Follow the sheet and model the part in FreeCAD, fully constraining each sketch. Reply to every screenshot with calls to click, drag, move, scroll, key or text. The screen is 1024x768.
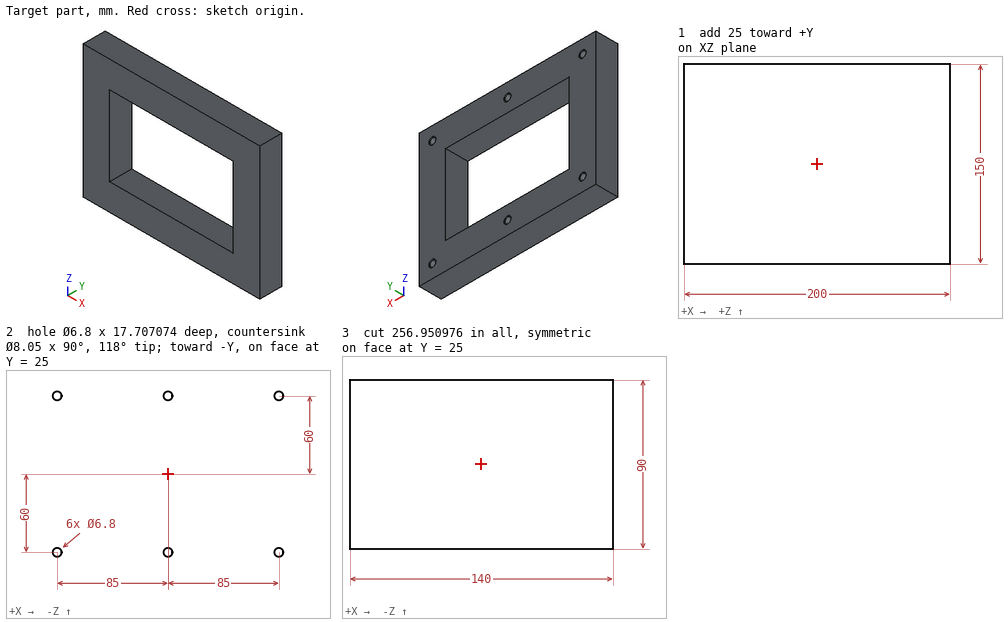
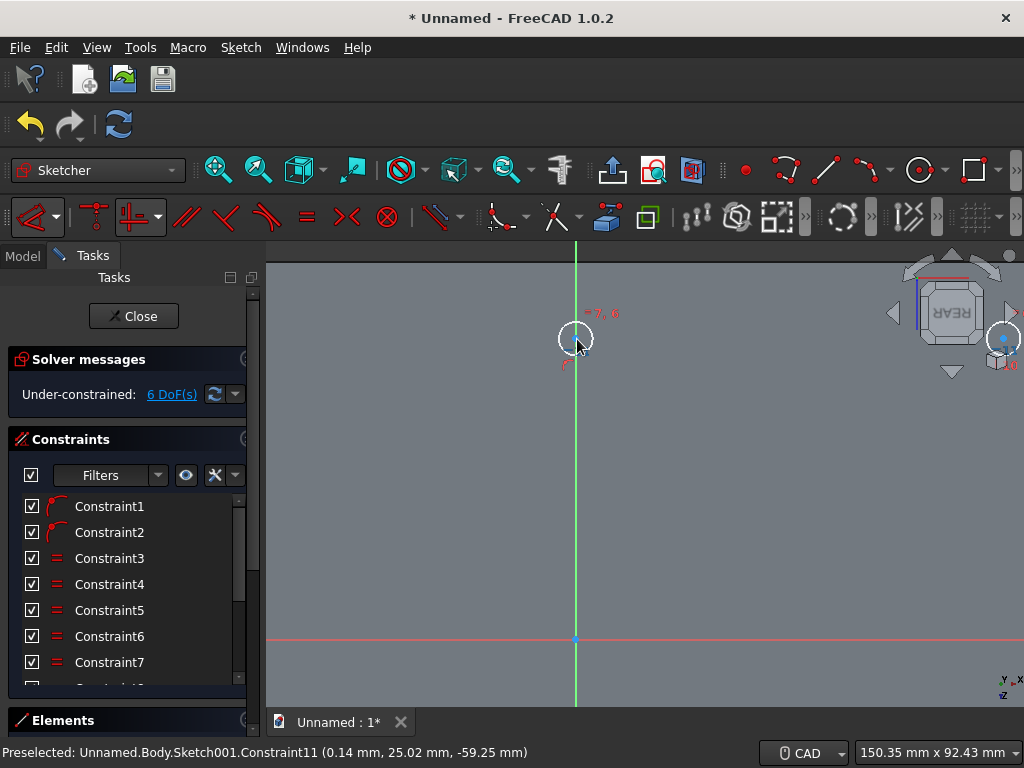
click(576, 339)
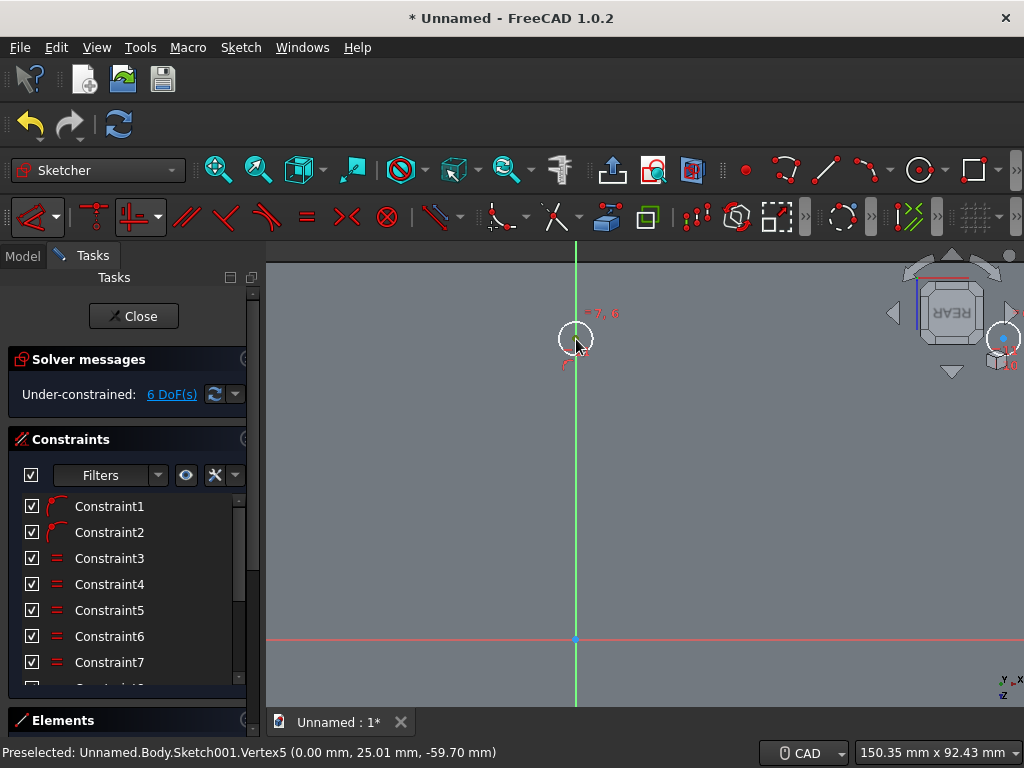
scroll(577, 339, down, 4)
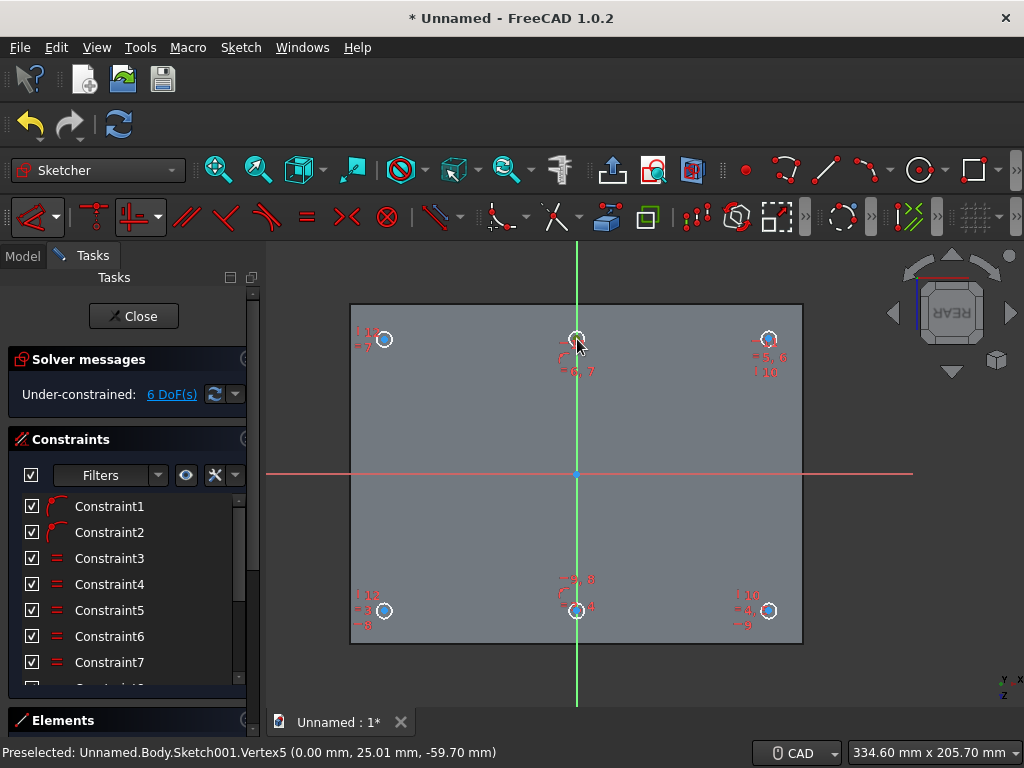
click(384, 339)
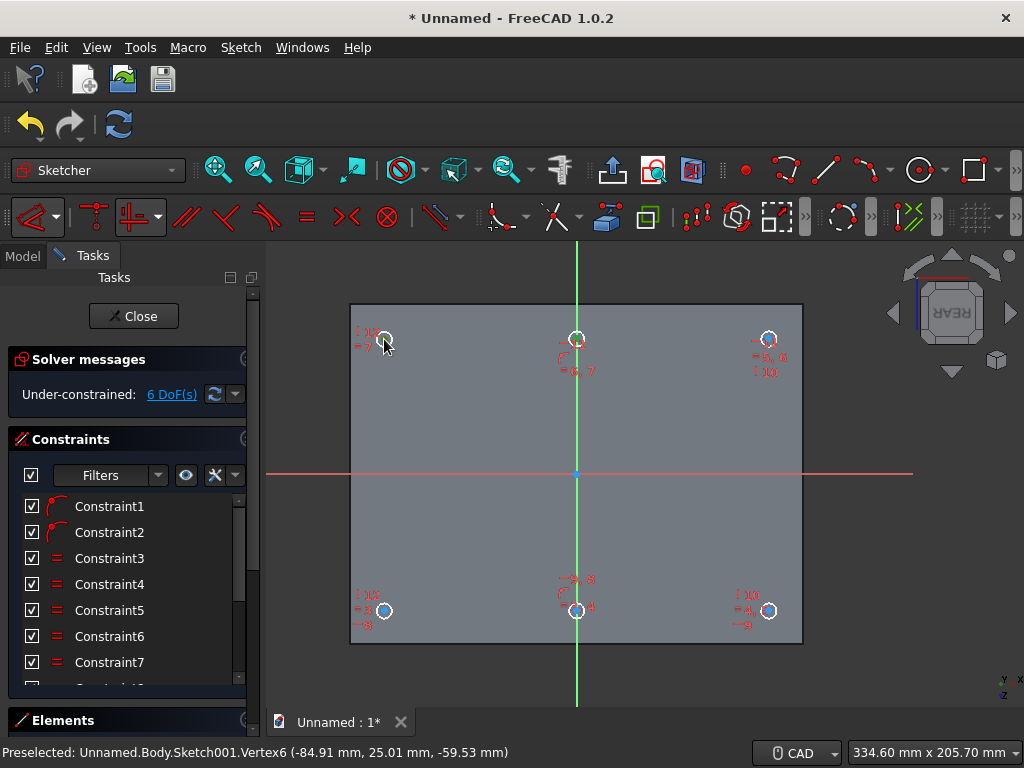
key(h)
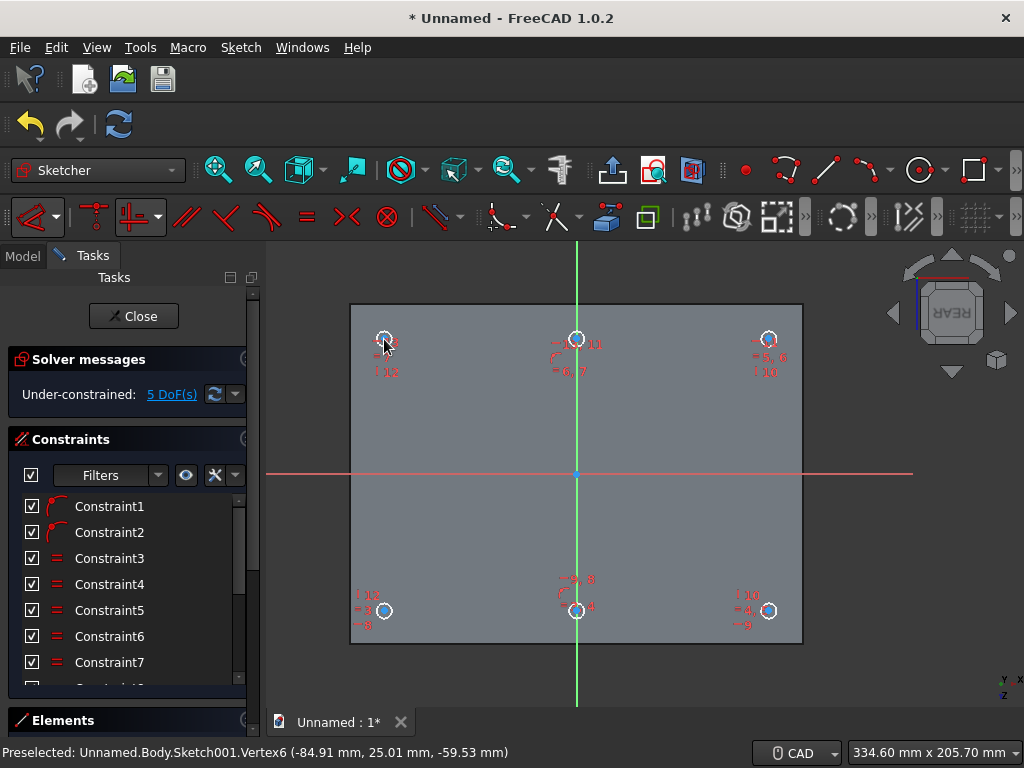
scroll(377, 611, up, 5)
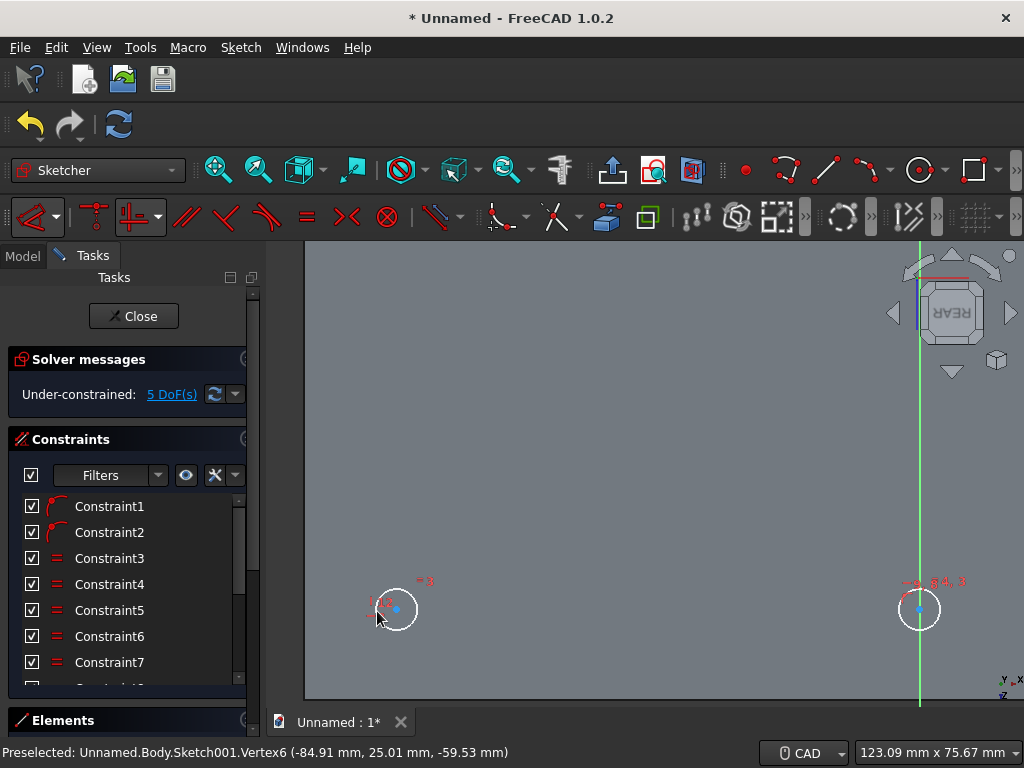
click(417, 610)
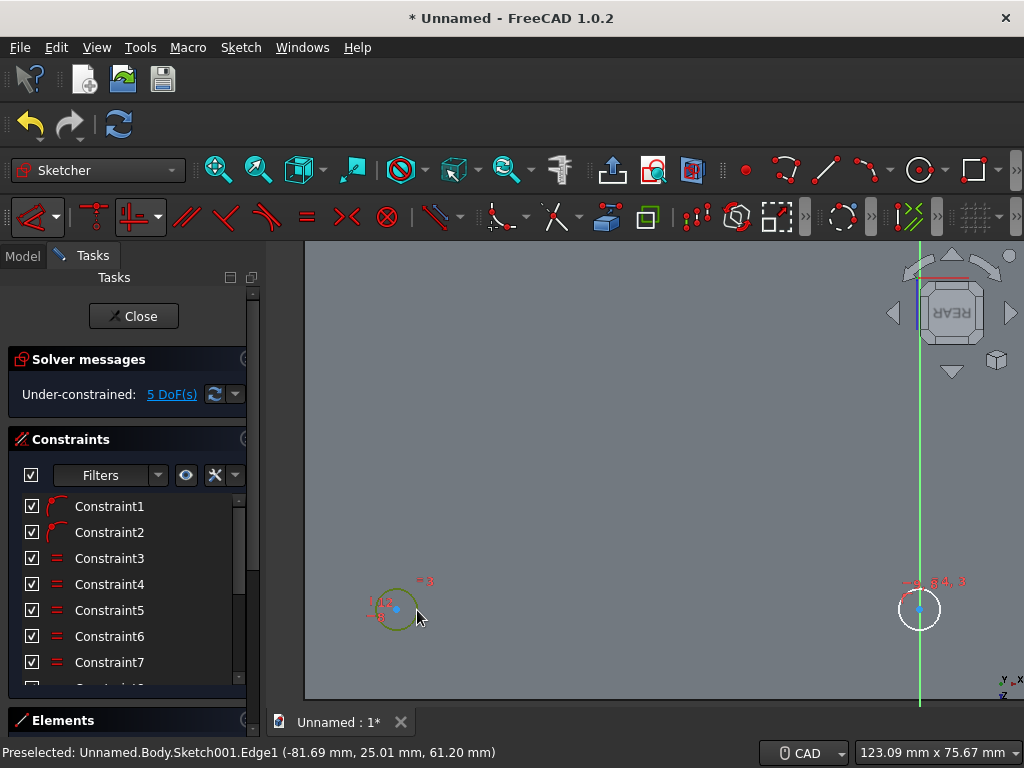
click(58, 218)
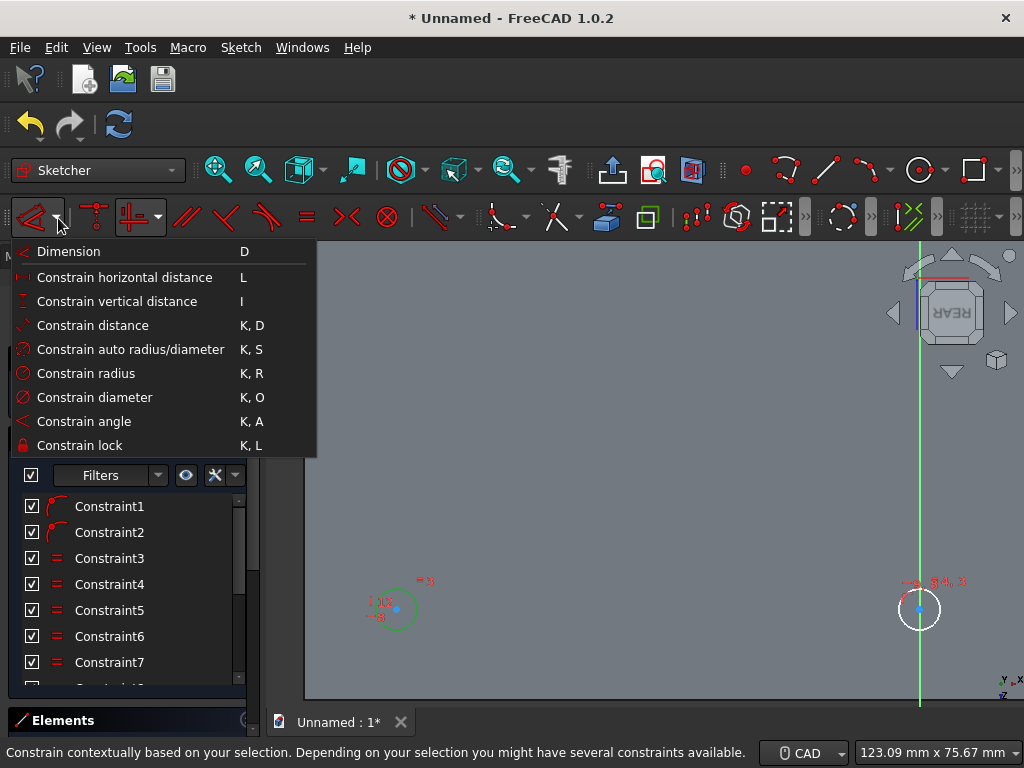
click(164, 397)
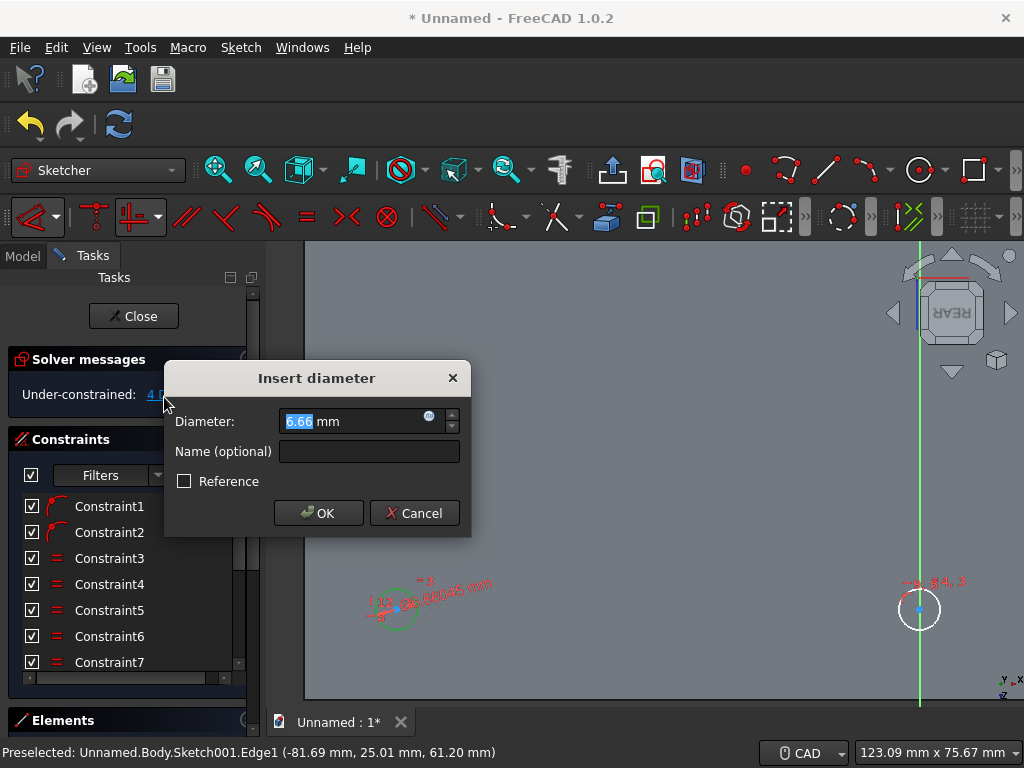
text(6.8)
key(Return)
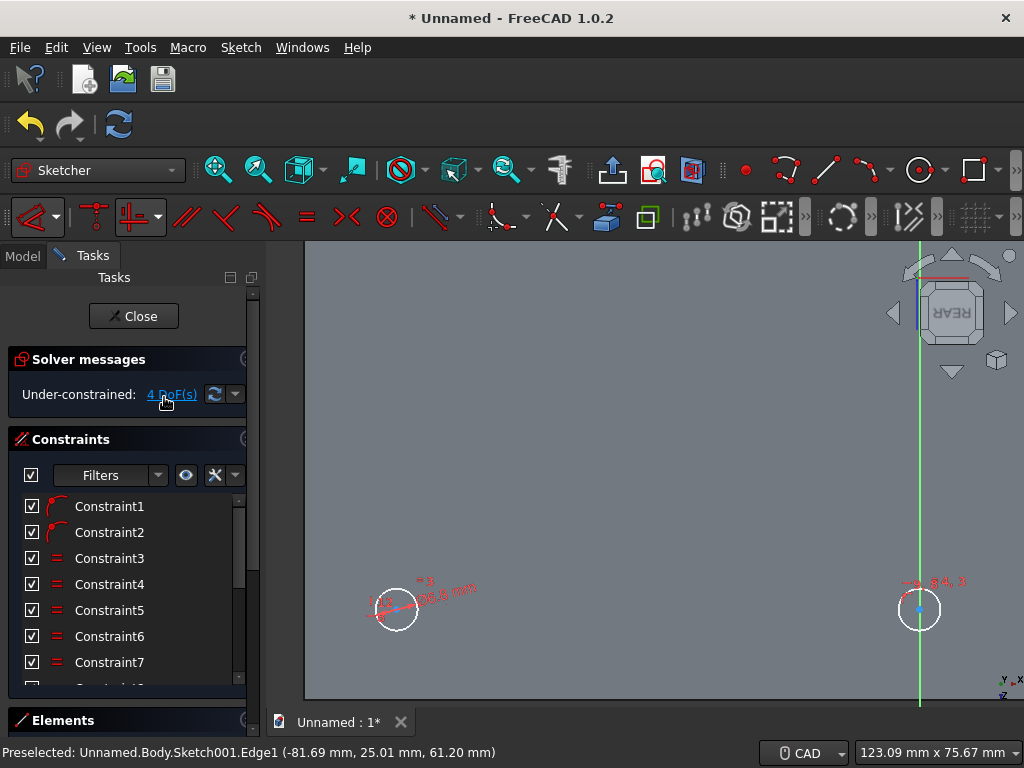
click(397, 610)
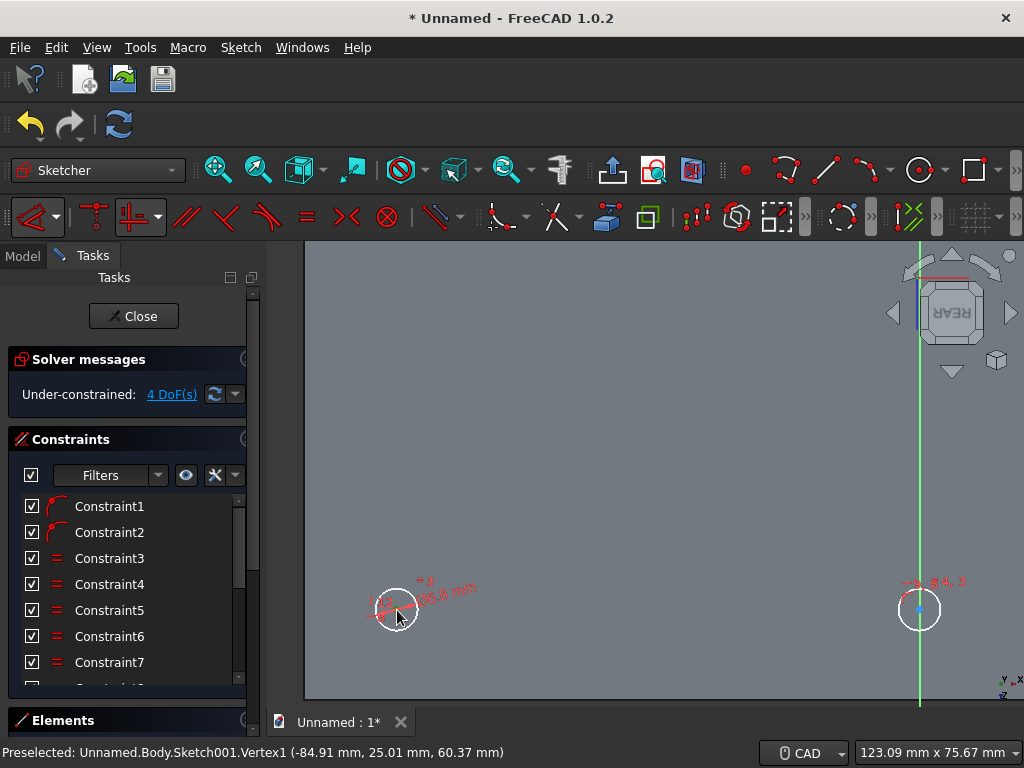
key(l)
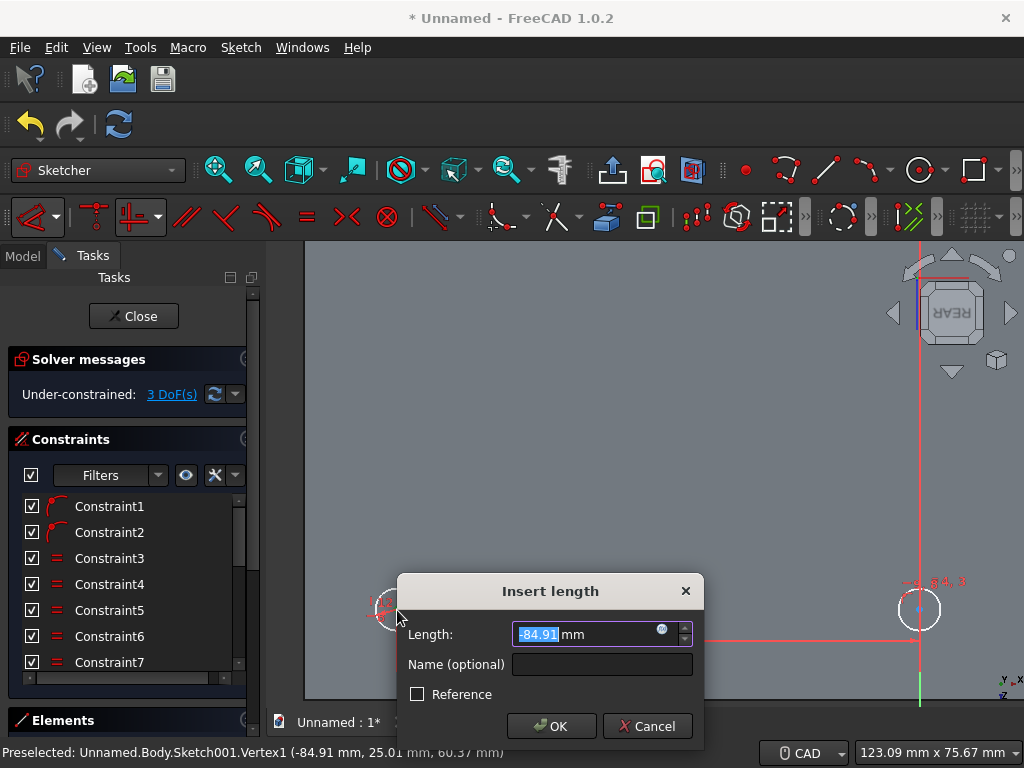
text(-85)
key(Return)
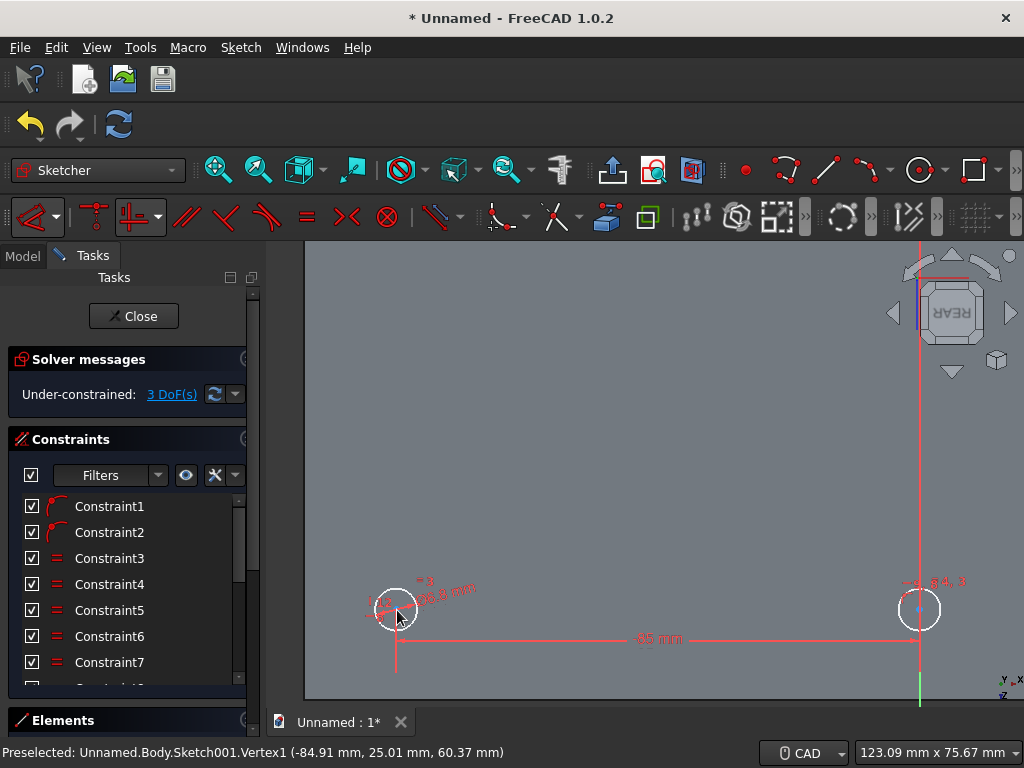
click(396, 610)